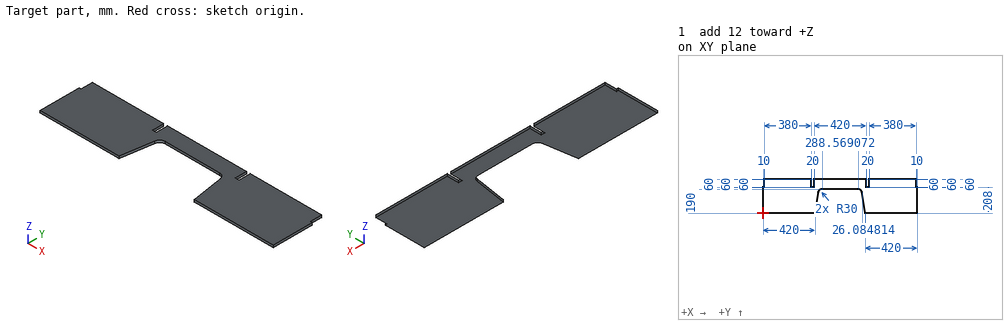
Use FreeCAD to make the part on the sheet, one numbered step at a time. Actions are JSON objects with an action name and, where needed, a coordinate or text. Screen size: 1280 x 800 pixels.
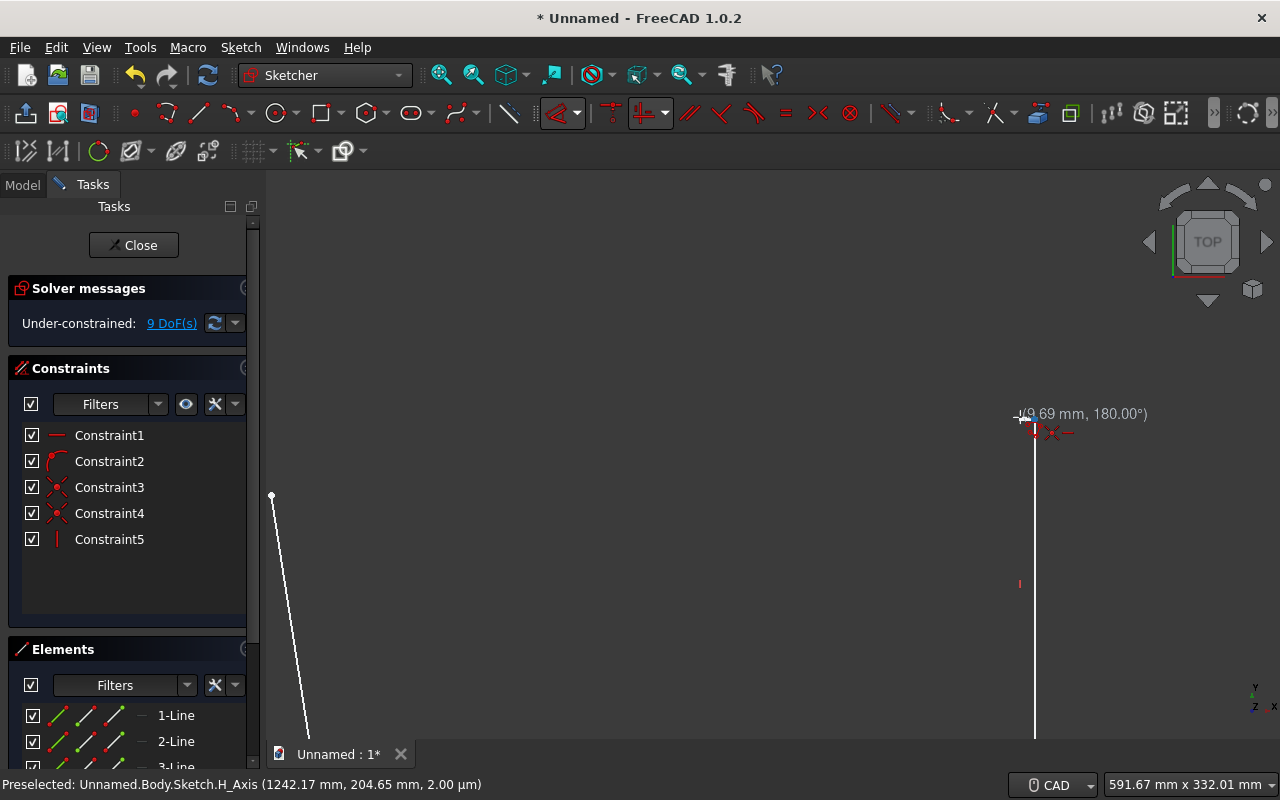
{"action": "left_click", "coordinate": [1017, 416]}
{"action": "left_click", "coordinate": [1017, 314]}
{"action": "left_click", "coordinate": [366, 314]}
{"action": "left_click", "coordinate": [366, 417]}
{"action": "left_click", "coordinate": [332, 417]}
{"action": "left_click", "coordinate": [332, 314]}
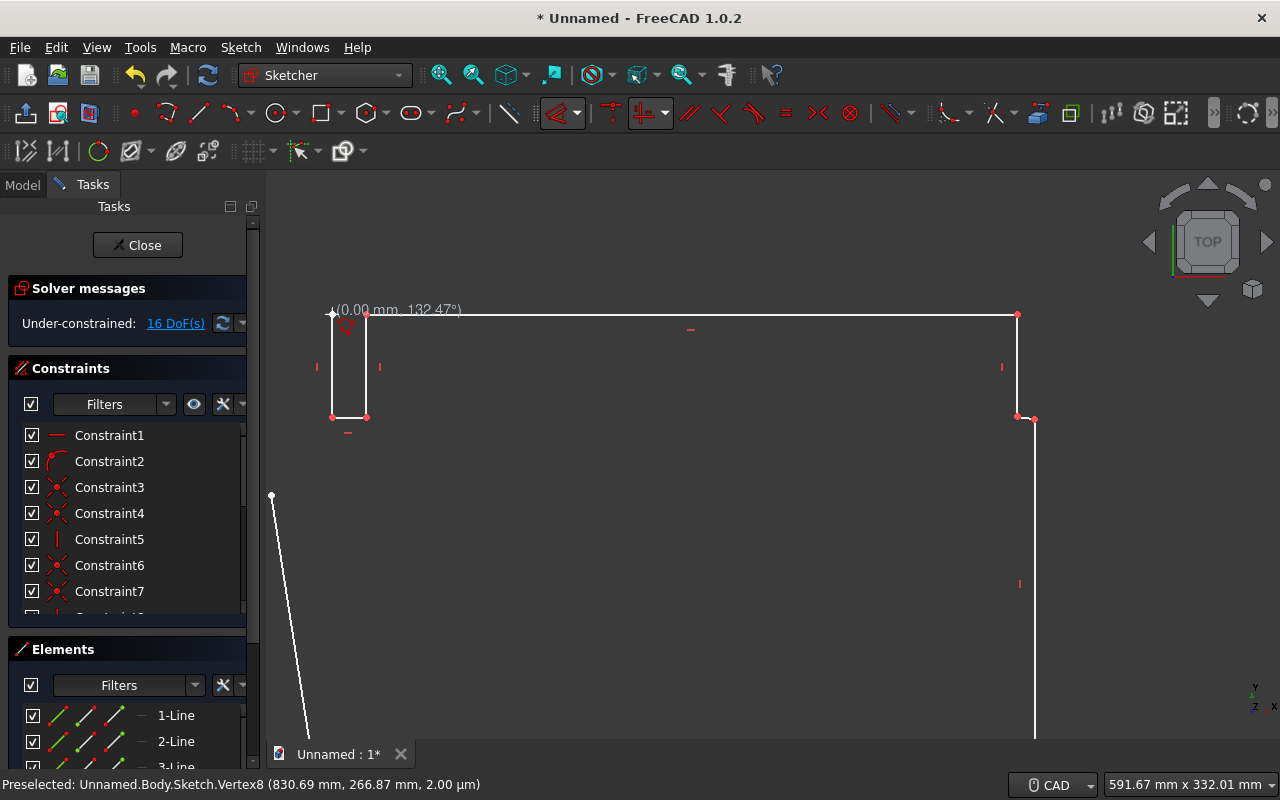
{"action": "scroll", "coordinate": [1020, 416], "scroll_direction": "down", "scroll_amount": 6}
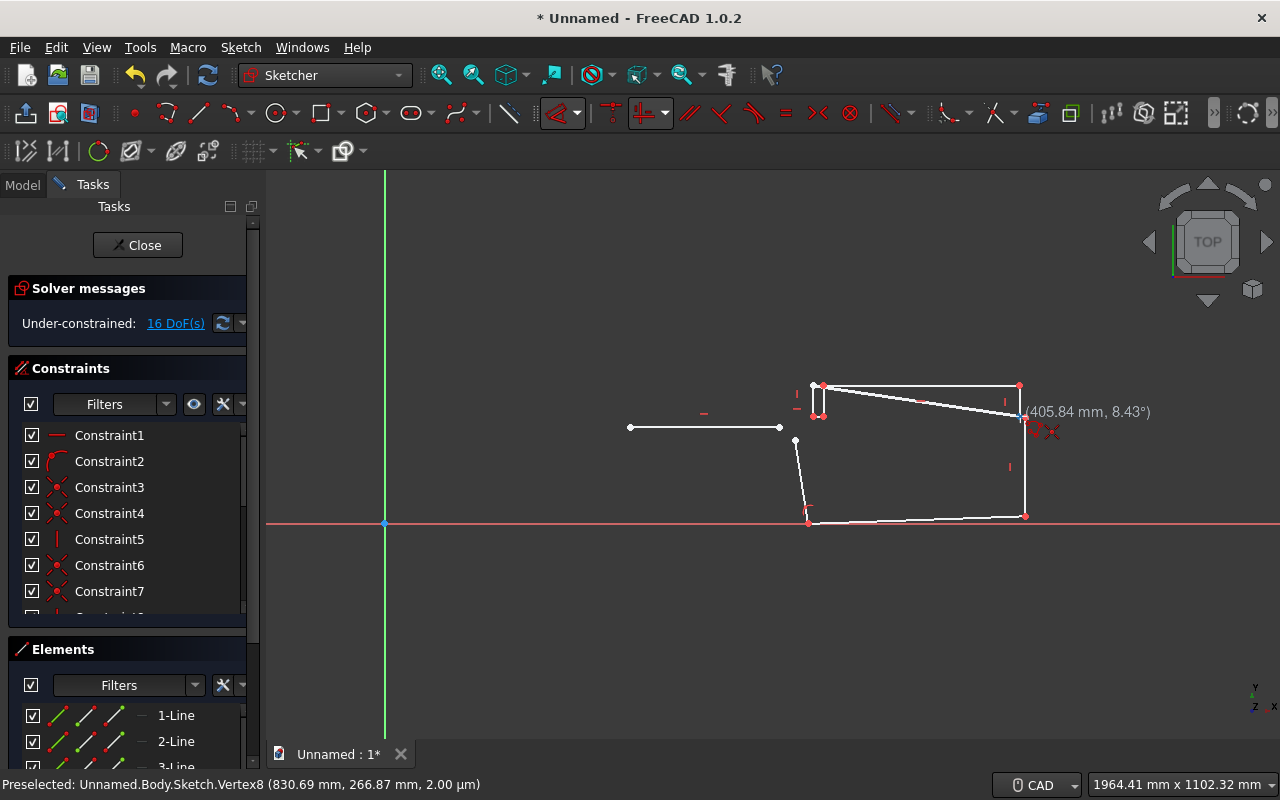
{"action": "left_click", "coordinate": [596, 386]}
{"action": "left_click", "coordinate": [596, 417]}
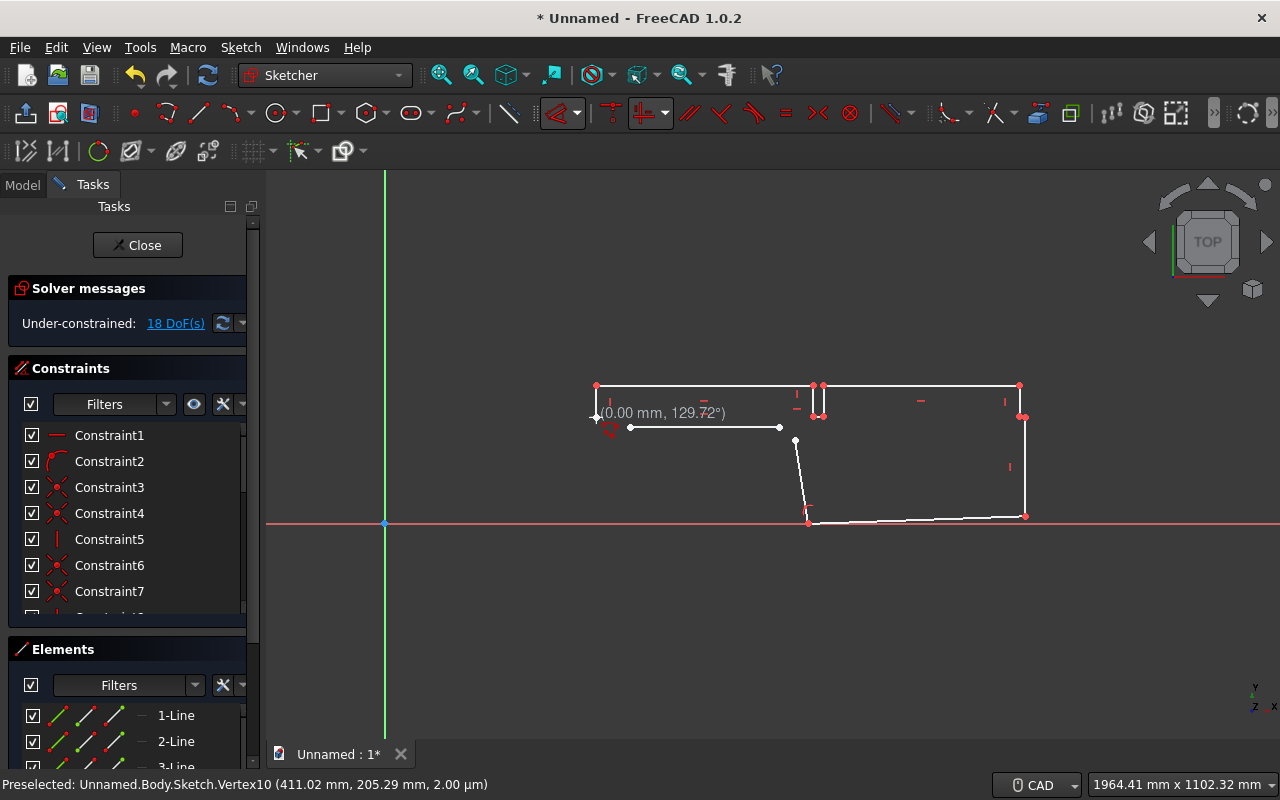
{"action": "scroll", "coordinate": [586, 417], "scroll_direction": "up", "scroll_amount": 3}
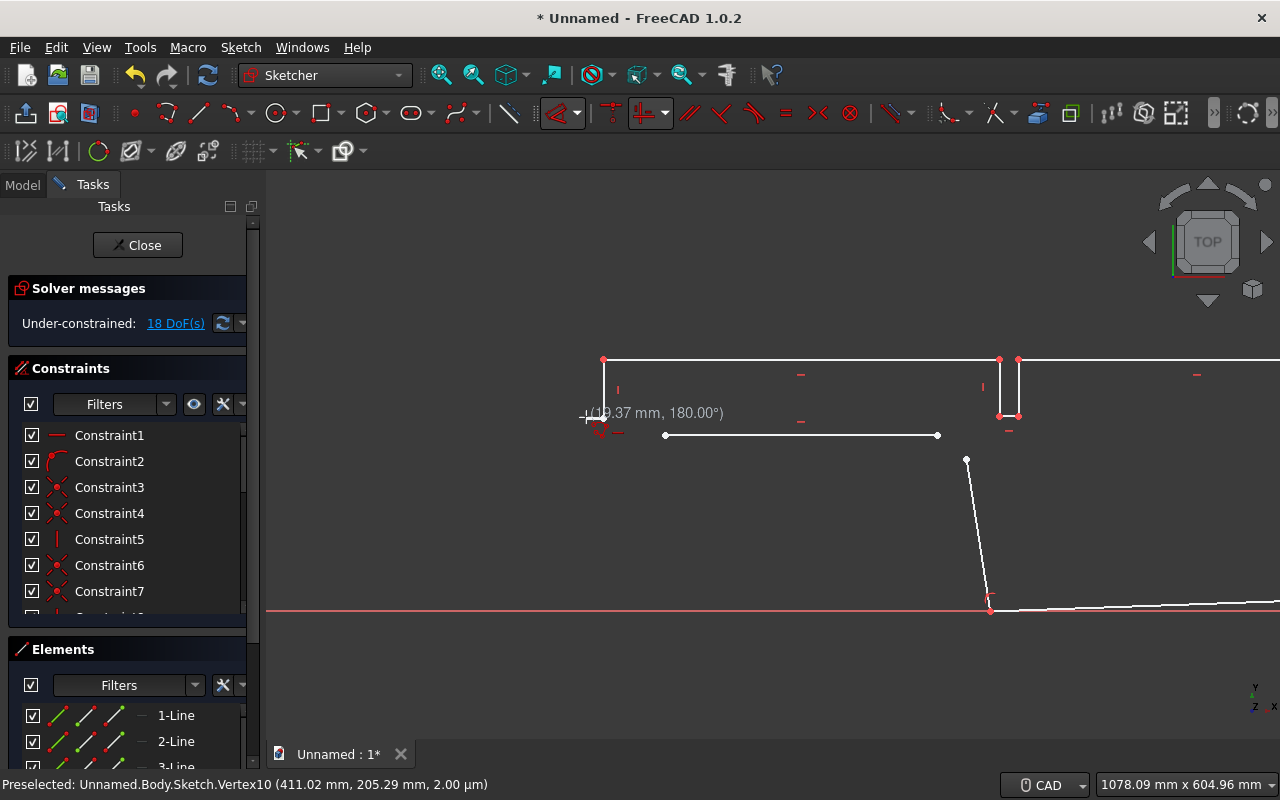
{"action": "left_click", "coordinate": [586, 417]}
{"action": "left_click", "coordinate": [586, 359]}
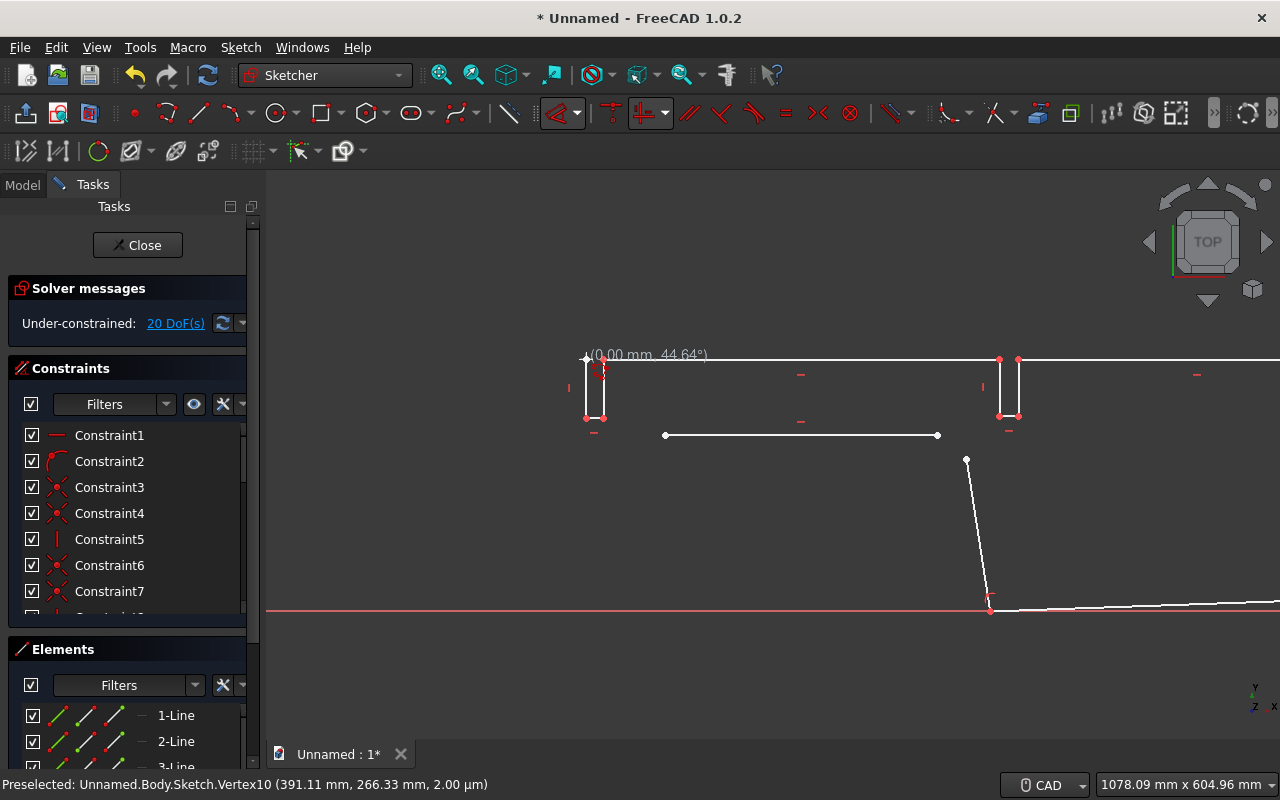
{"action": "scroll", "coordinate": [586, 417], "scroll_direction": "down", "scroll_amount": 3}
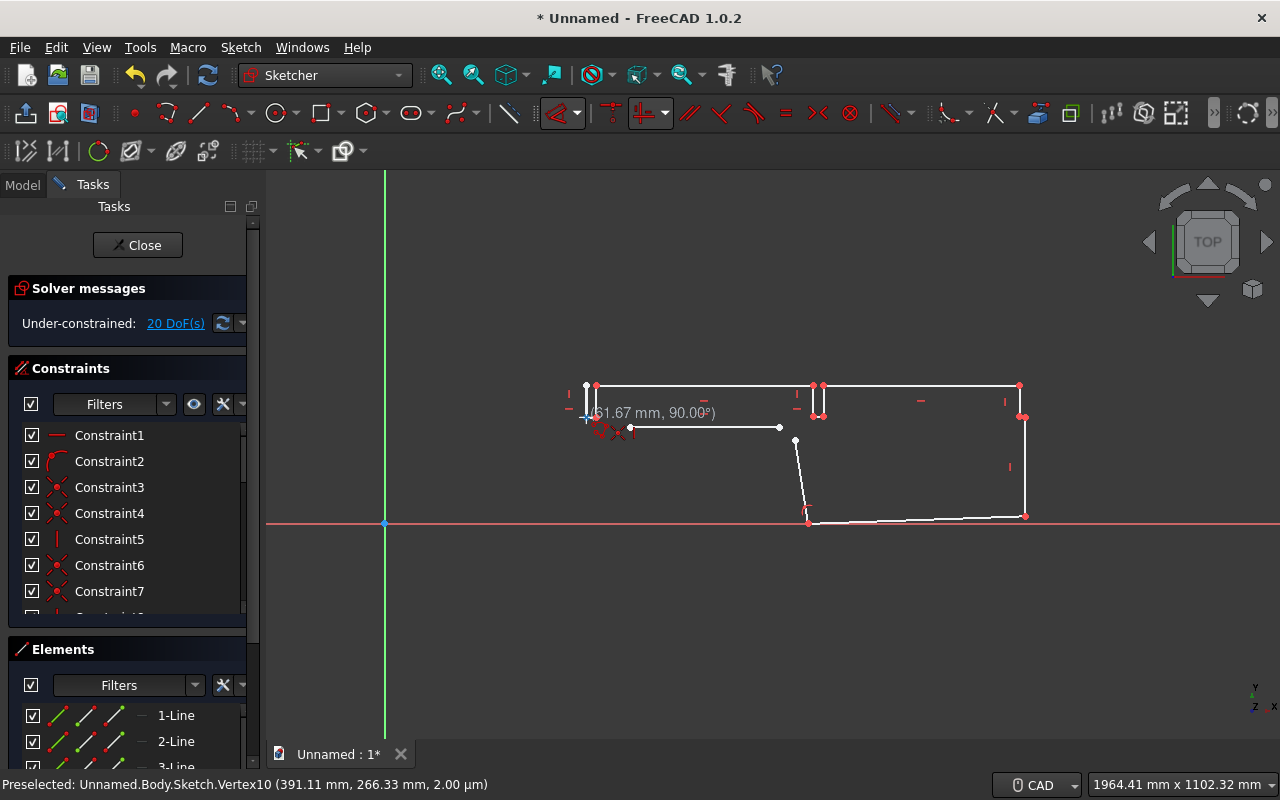
{"action": "scroll", "coordinate": [390, 386], "scroll_direction": "up", "scroll_amount": 6}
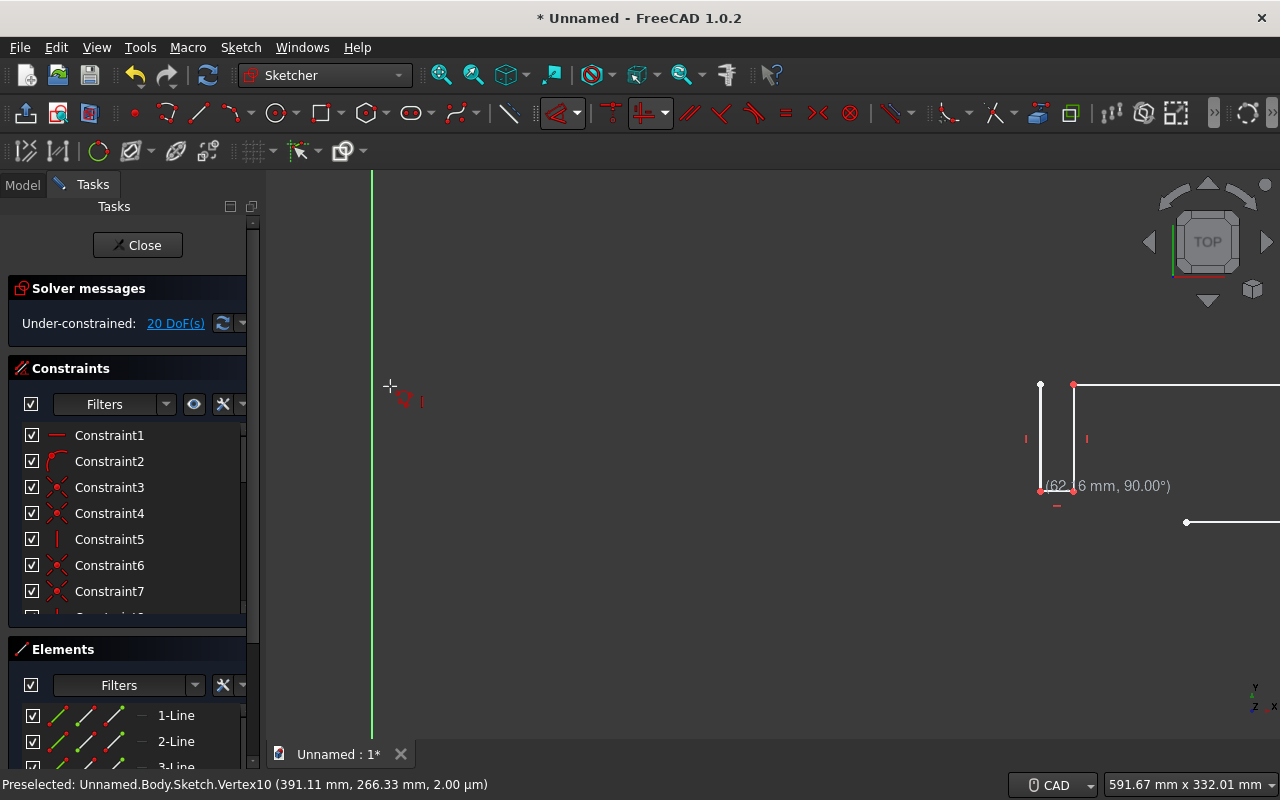
{"action": "left_click", "coordinate": [390, 383]}
{"action": "left_click", "coordinate": [390, 487]}
{"action": "left_click", "coordinate": [372, 487]}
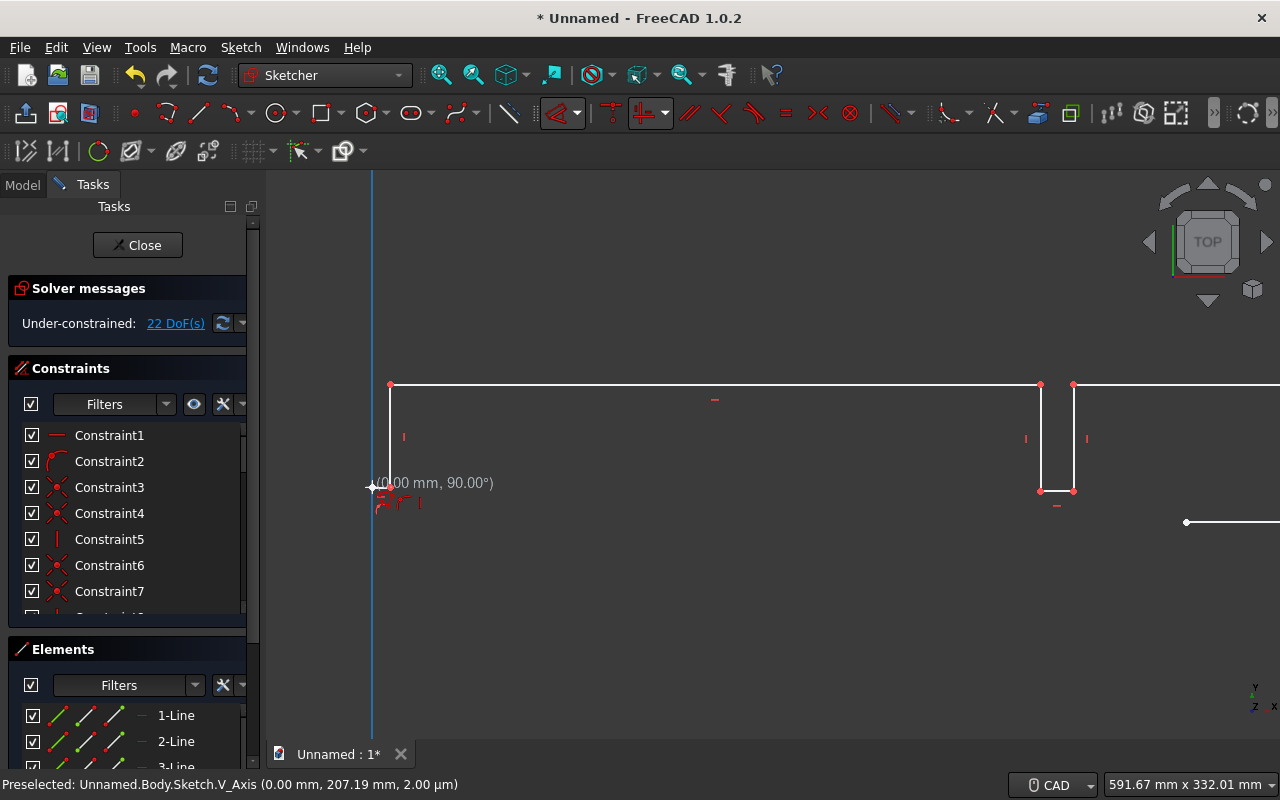
{"action": "scroll", "coordinate": [390, 386], "scroll_direction": "down", "scroll_amount": 6}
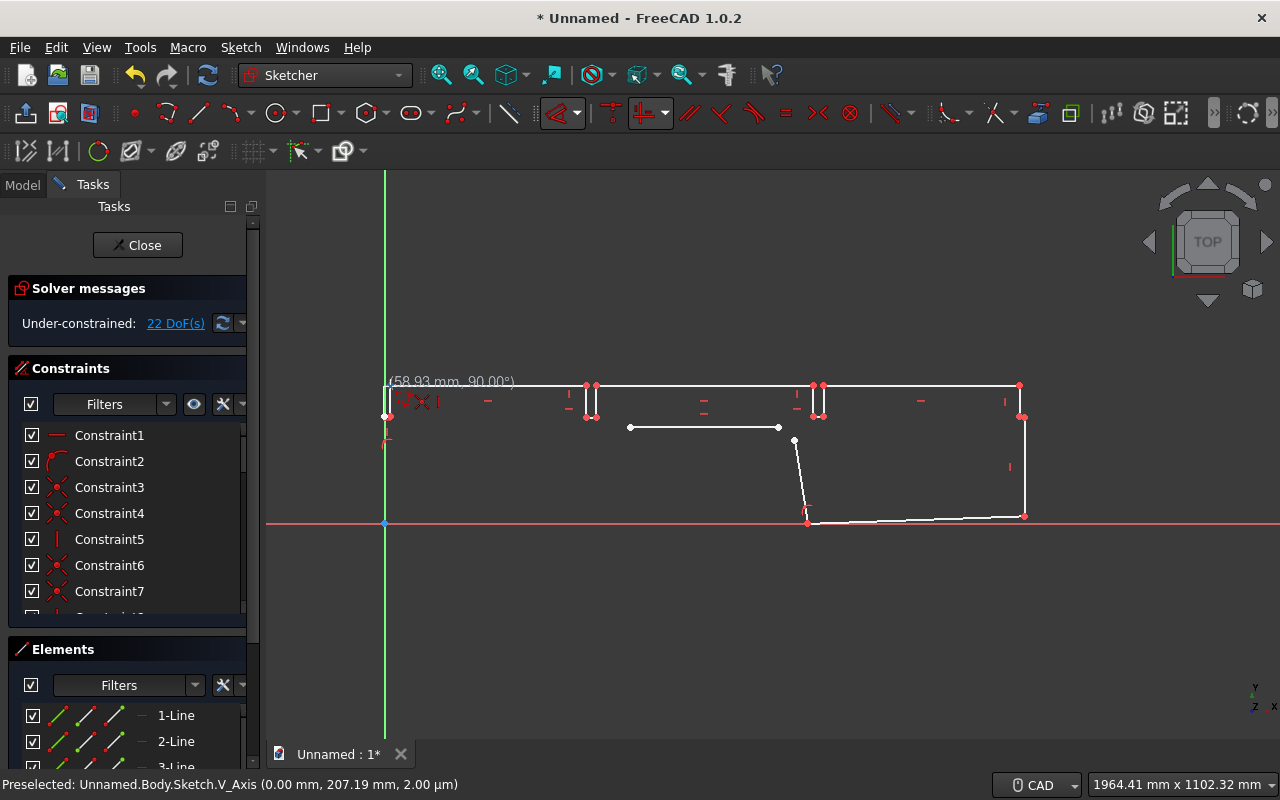
{"action": "left_click", "coordinate": [385, 524]}
{"action": "left_click", "coordinate": [602, 515]}
{"action": "left_click", "coordinate": [615, 439]}
{"action": "right_click", "coordinate": [615, 439]}